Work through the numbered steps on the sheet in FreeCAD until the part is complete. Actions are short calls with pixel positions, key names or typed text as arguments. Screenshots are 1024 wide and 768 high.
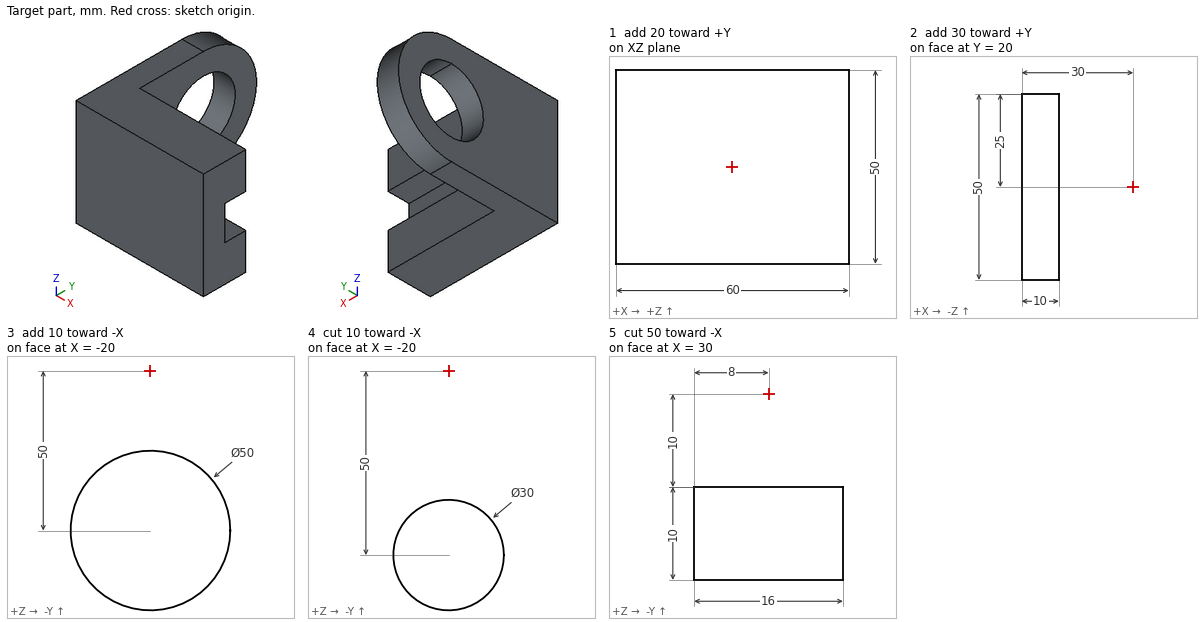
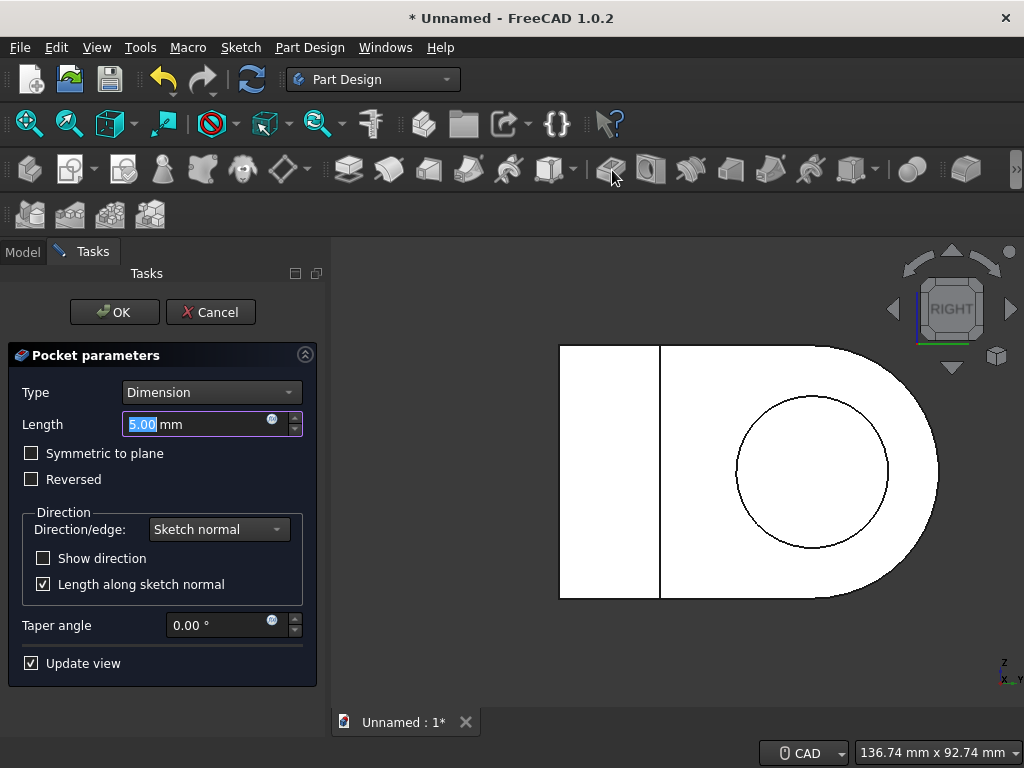
text(10)
key(Tab)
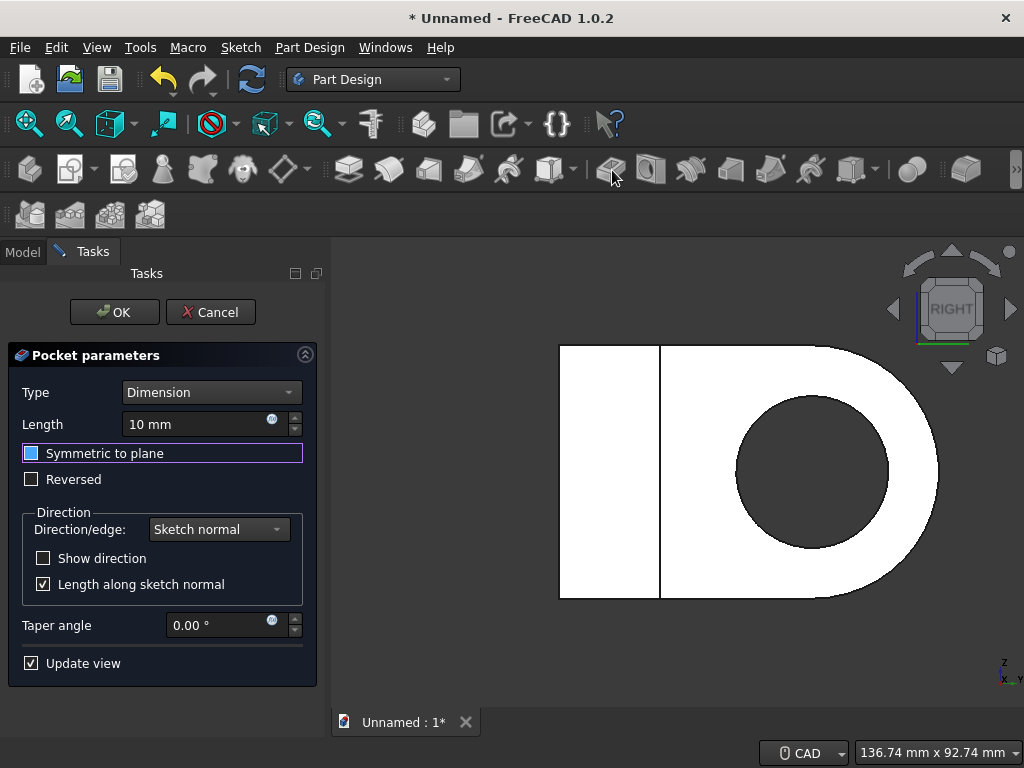
click(115, 312)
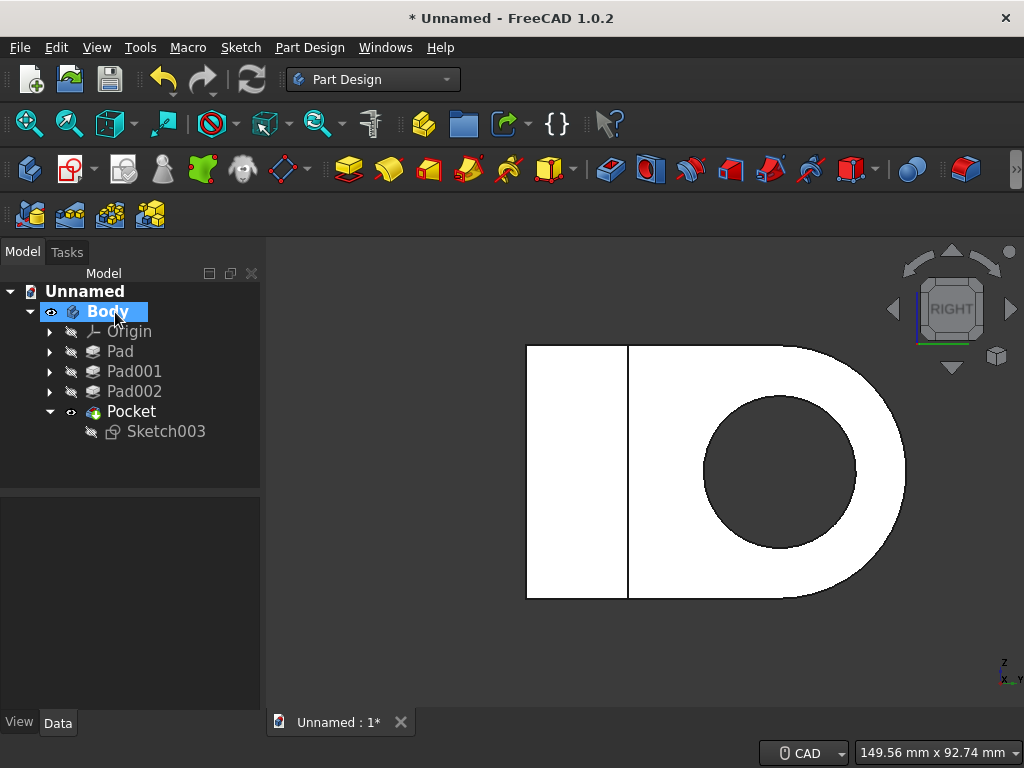
click(577, 471)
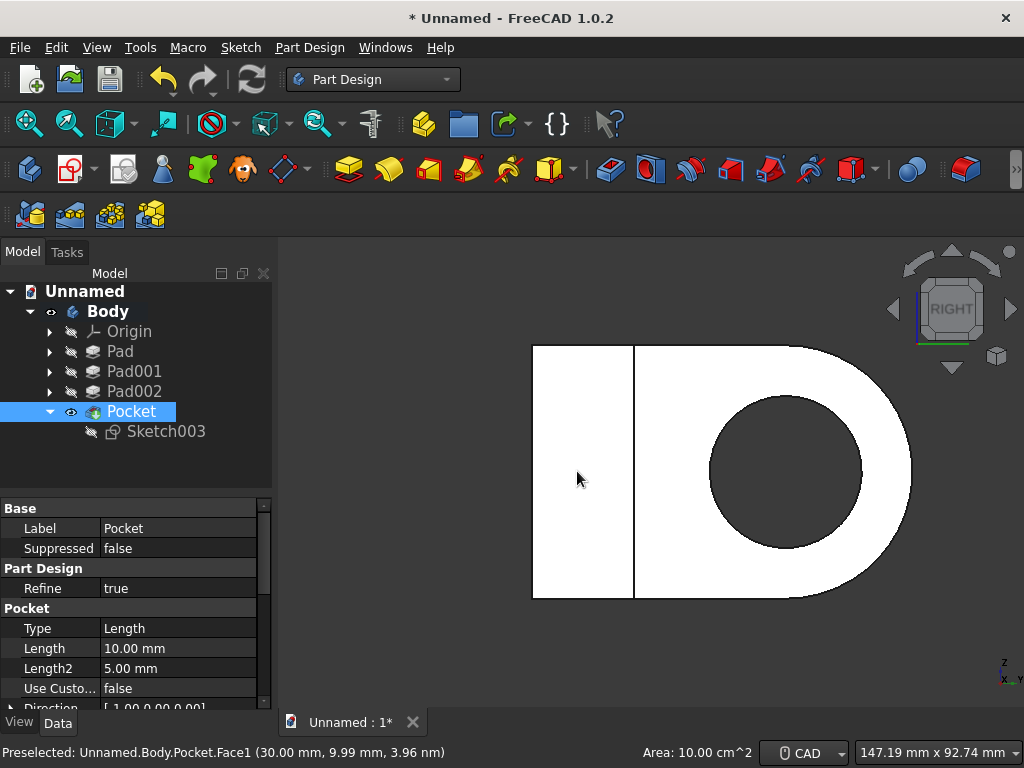
click(70, 170)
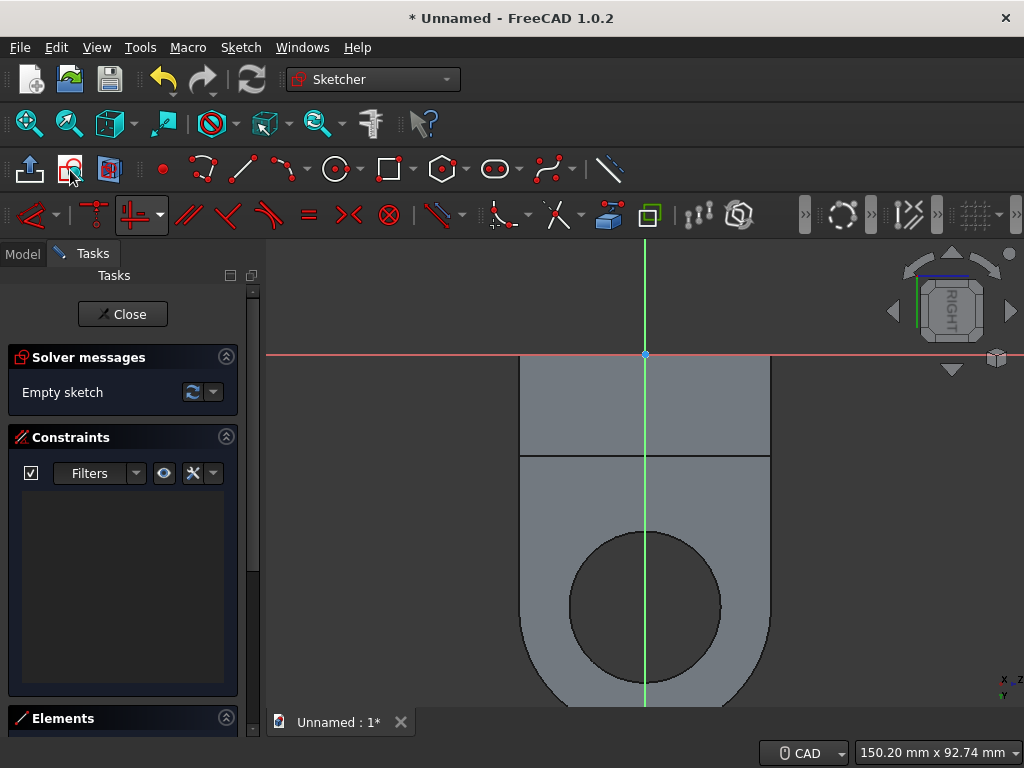
scroll(685, 366, up, 5)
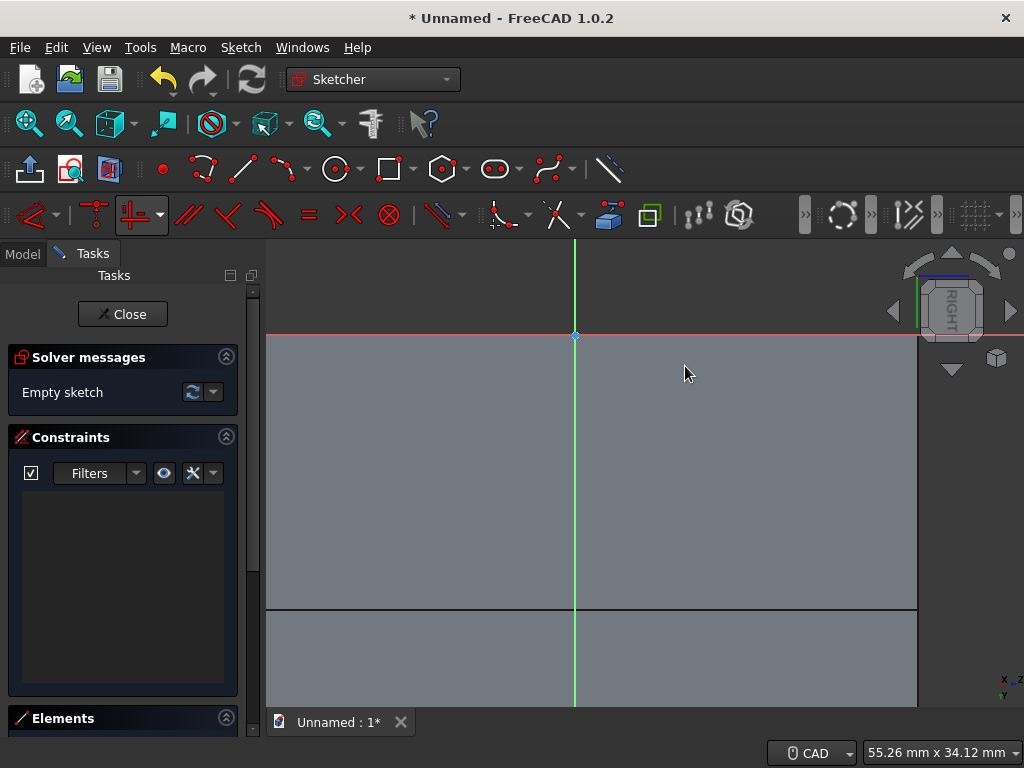
click(390, 170)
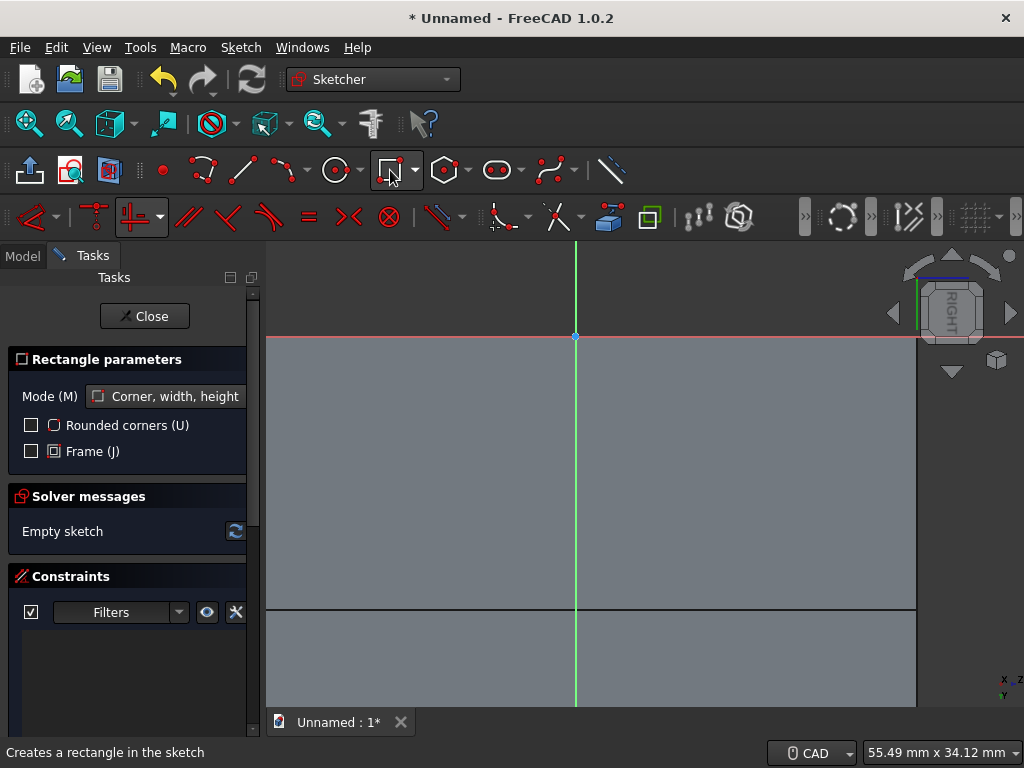
click(466, 473)
click(685, 610)
key(Escape)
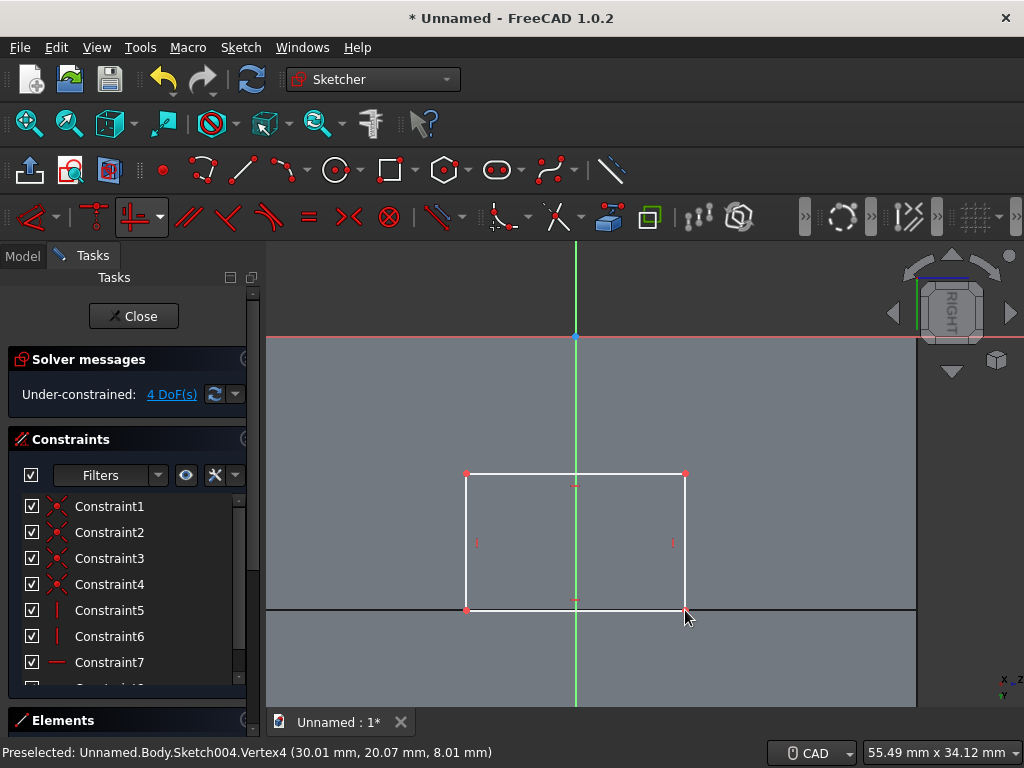
click(32, 218)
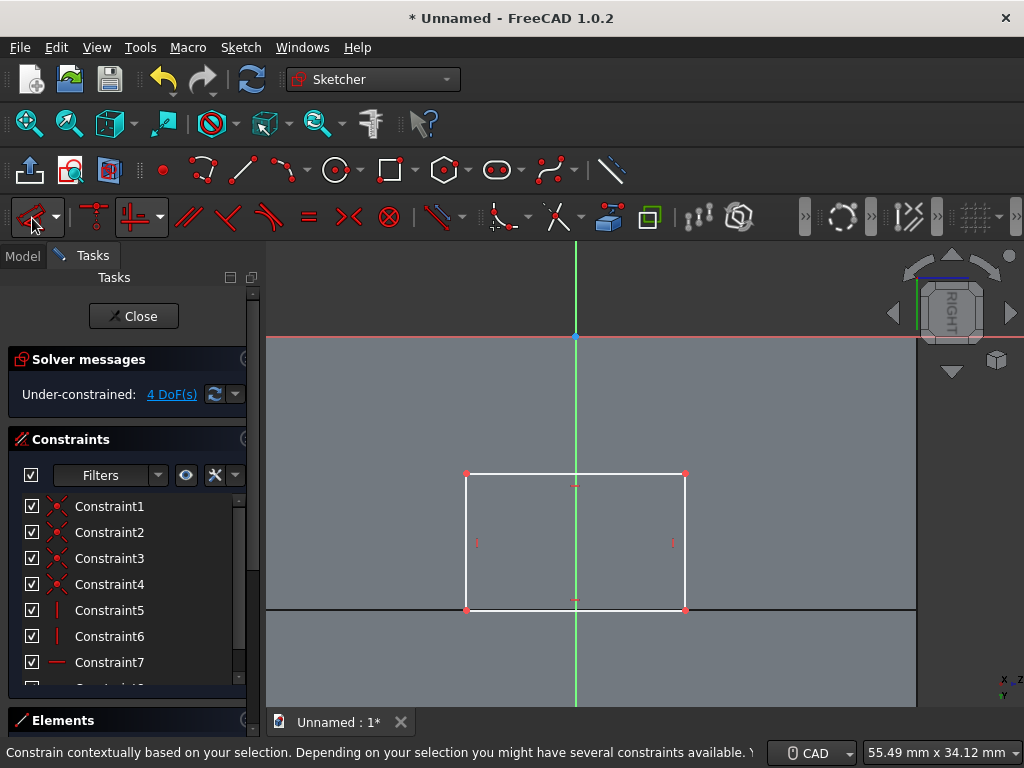
click(466, 515)
click(432, 543)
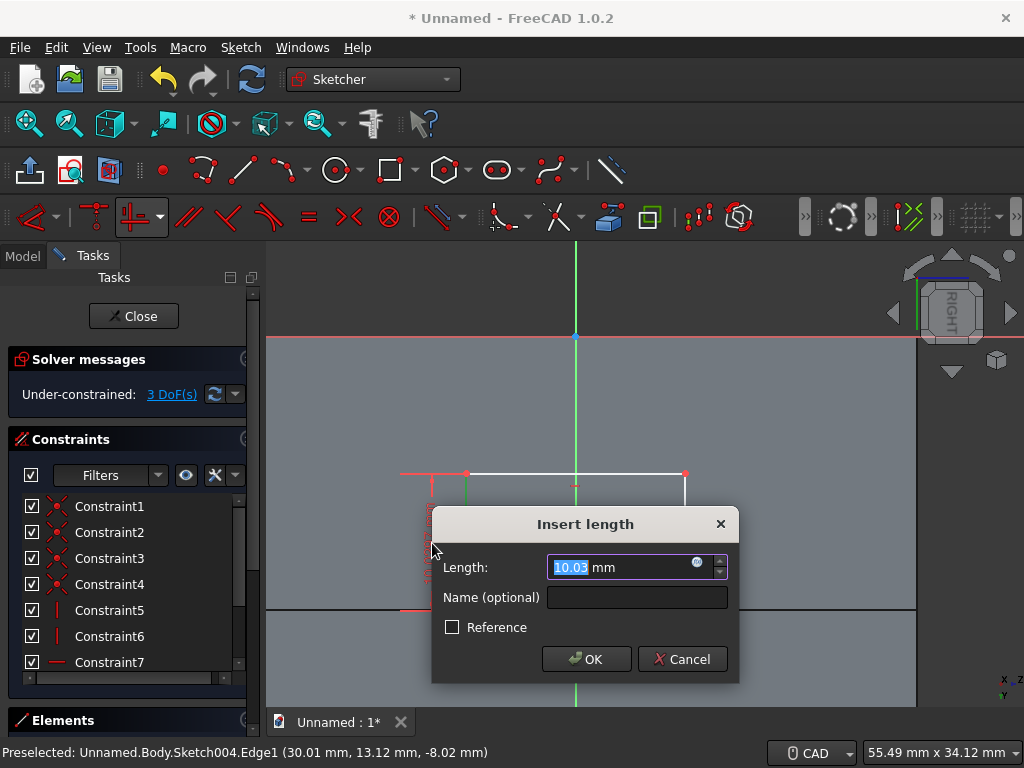
text(10)
key(Return)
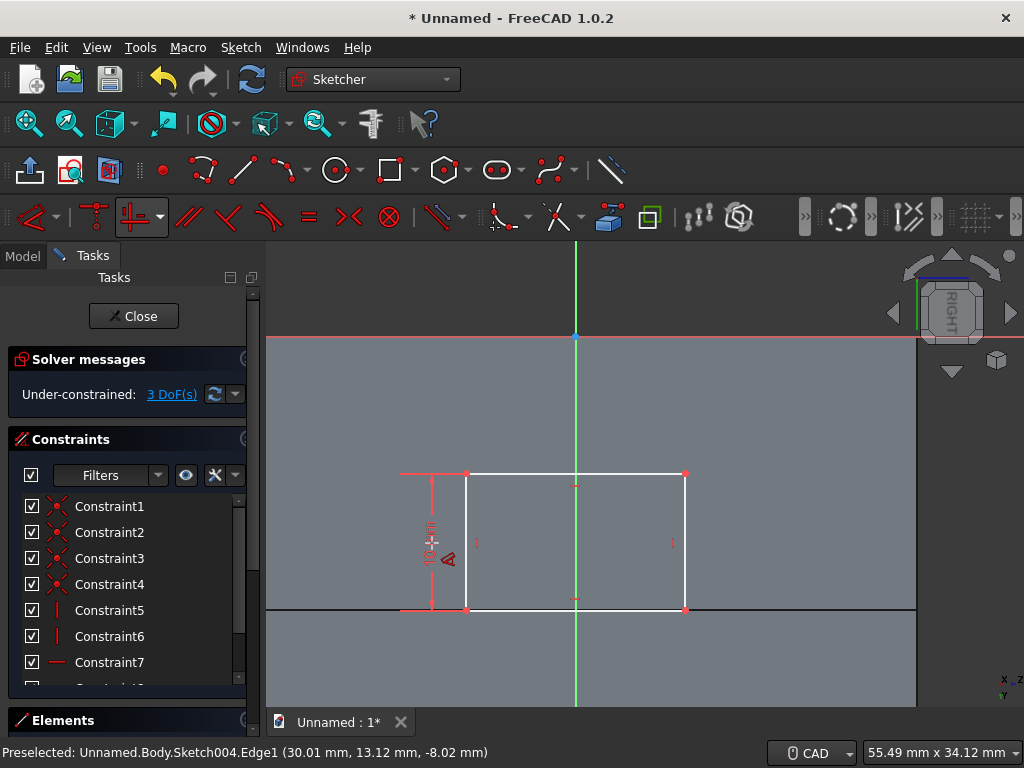
click(532, 611)
click(525, 645)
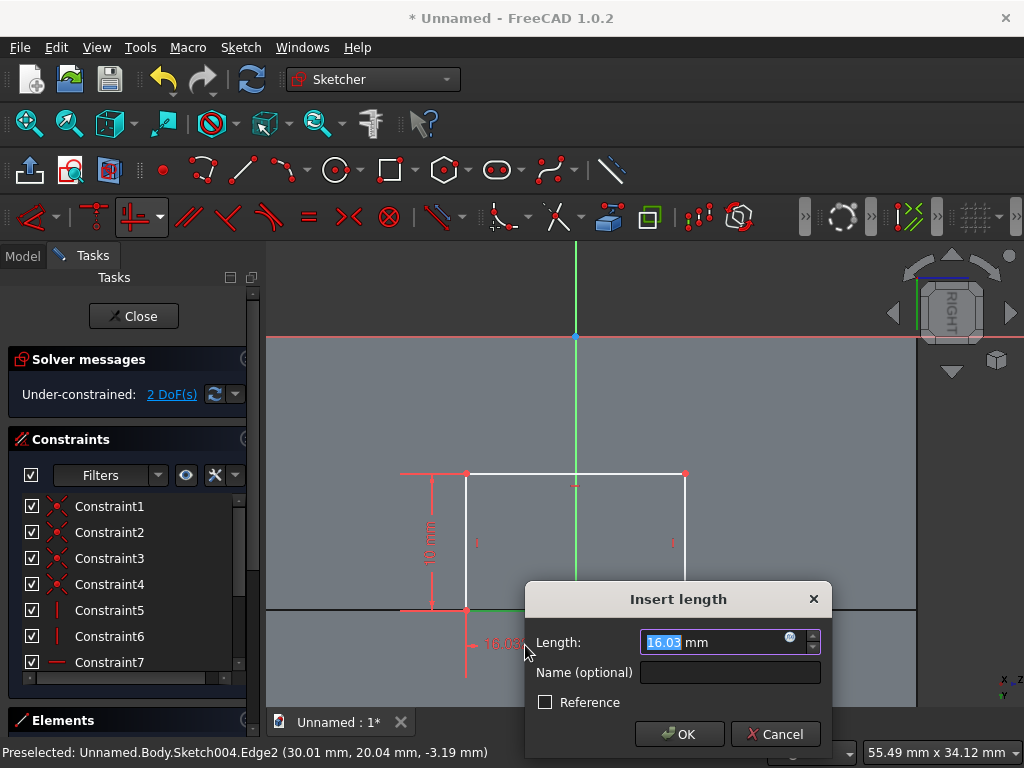
text(16)
key(Return)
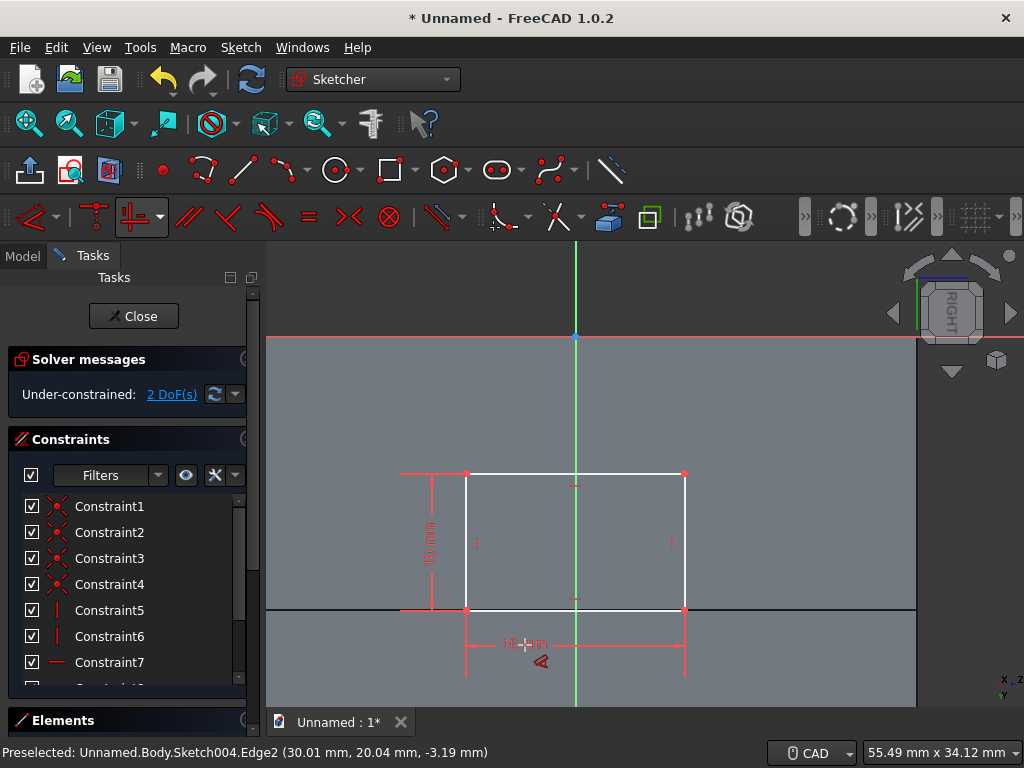
click(466, 474)
click(521, 303)